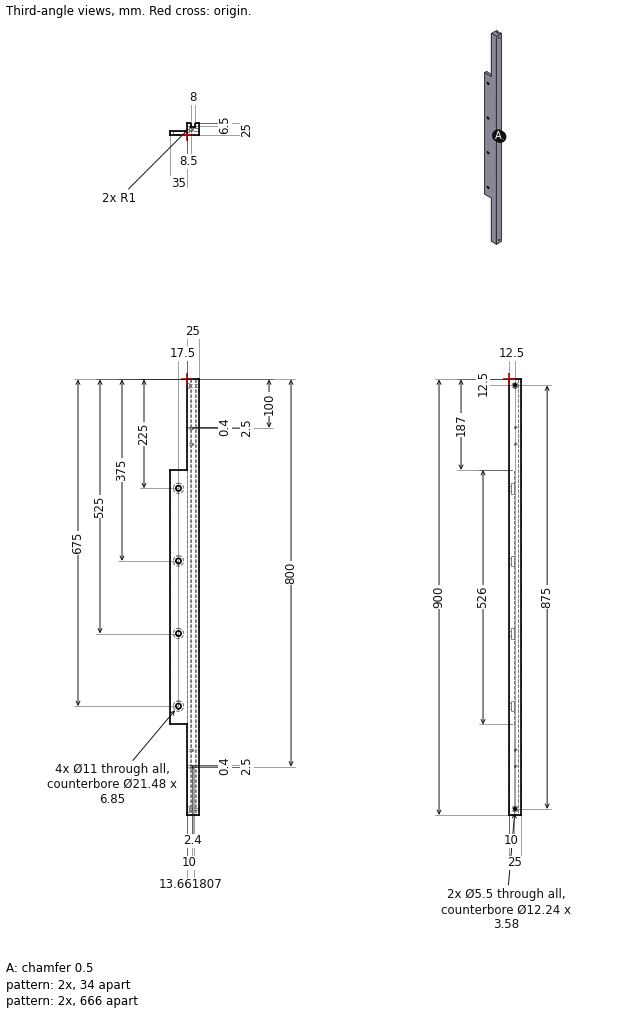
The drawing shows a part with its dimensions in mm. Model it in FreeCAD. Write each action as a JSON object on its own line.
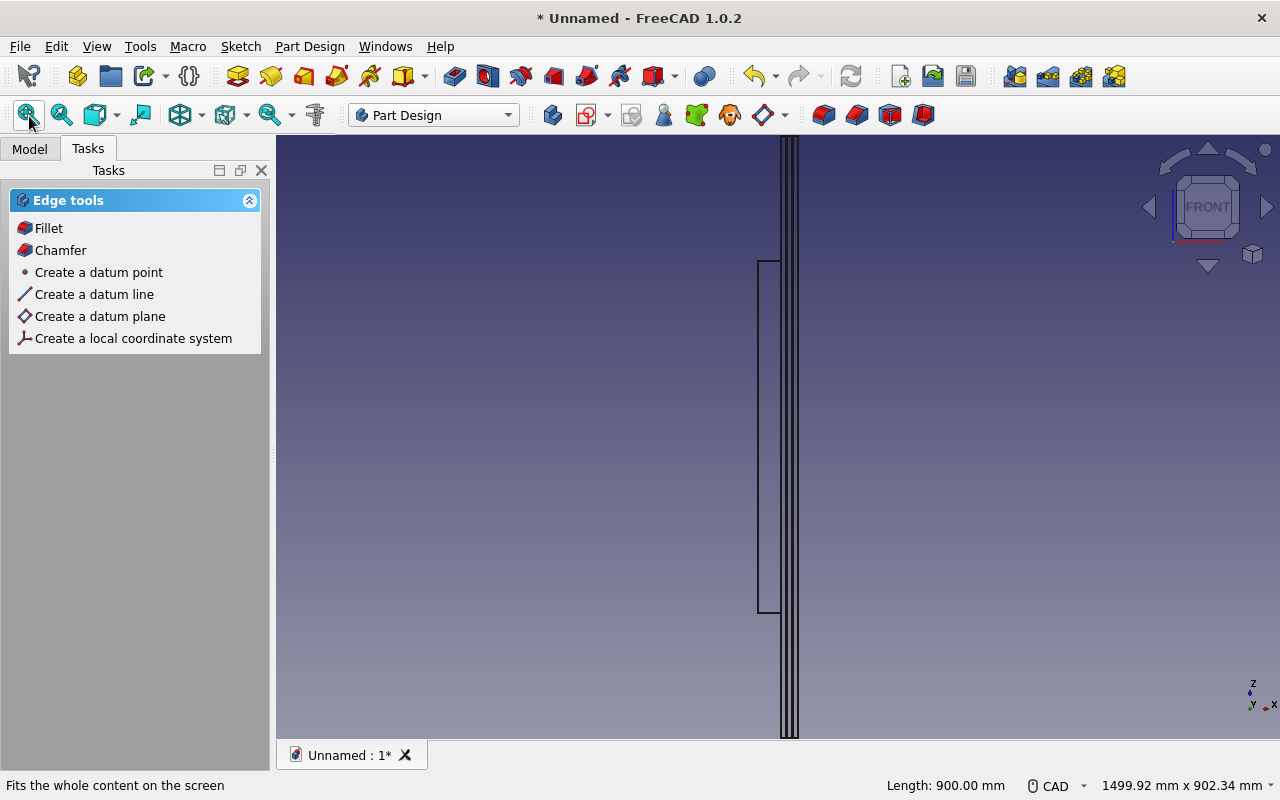
{"action": "key", "text": "3"}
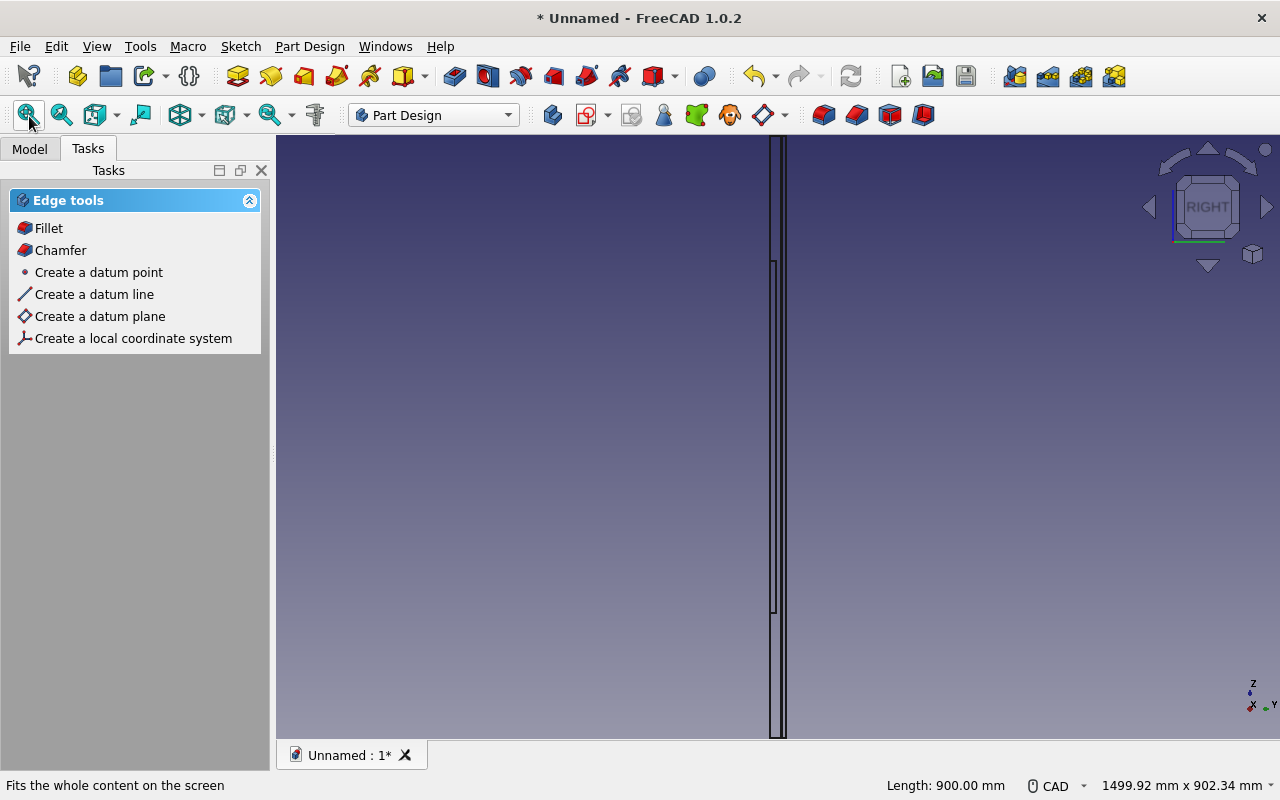
{"action": "scroll", "coordinate": [786, 436], "scroll_direction": "up", "scroll_amount": 6}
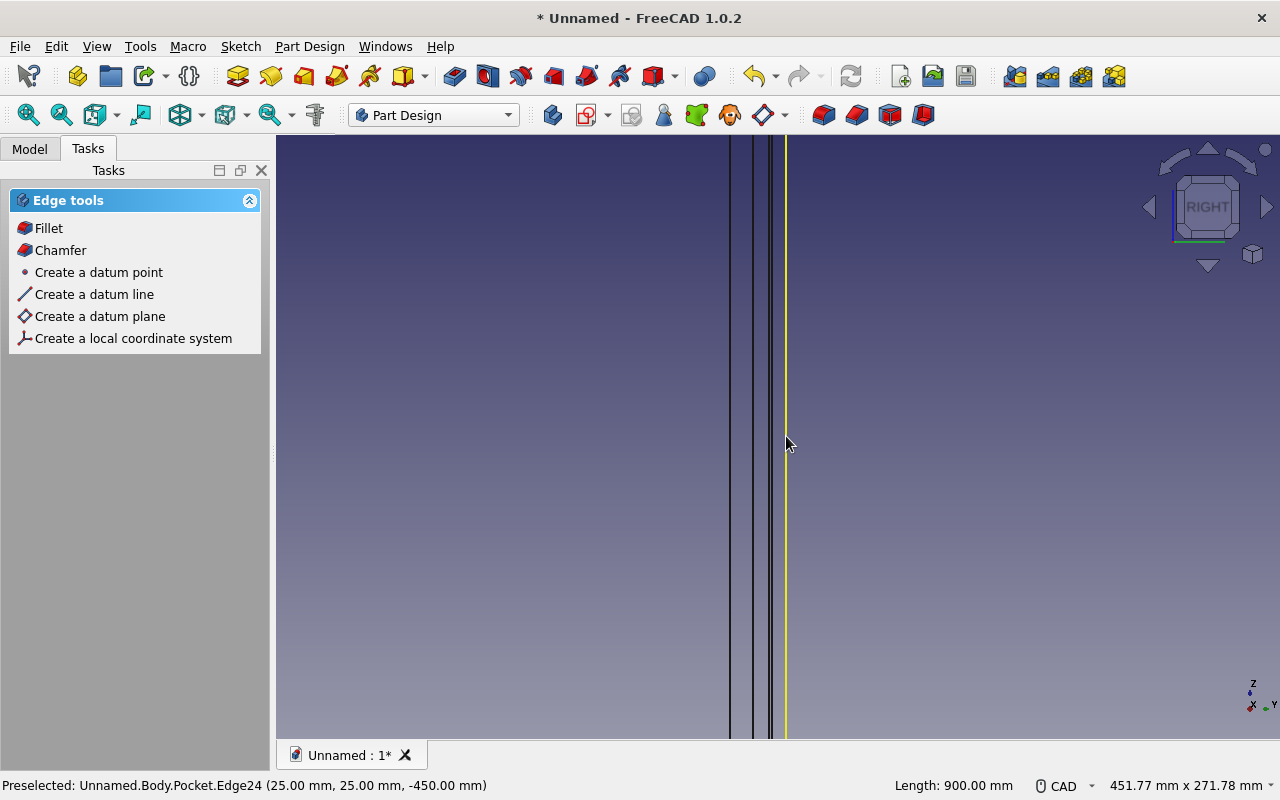
{"action": "left_click", "coordinate": [29, 116]}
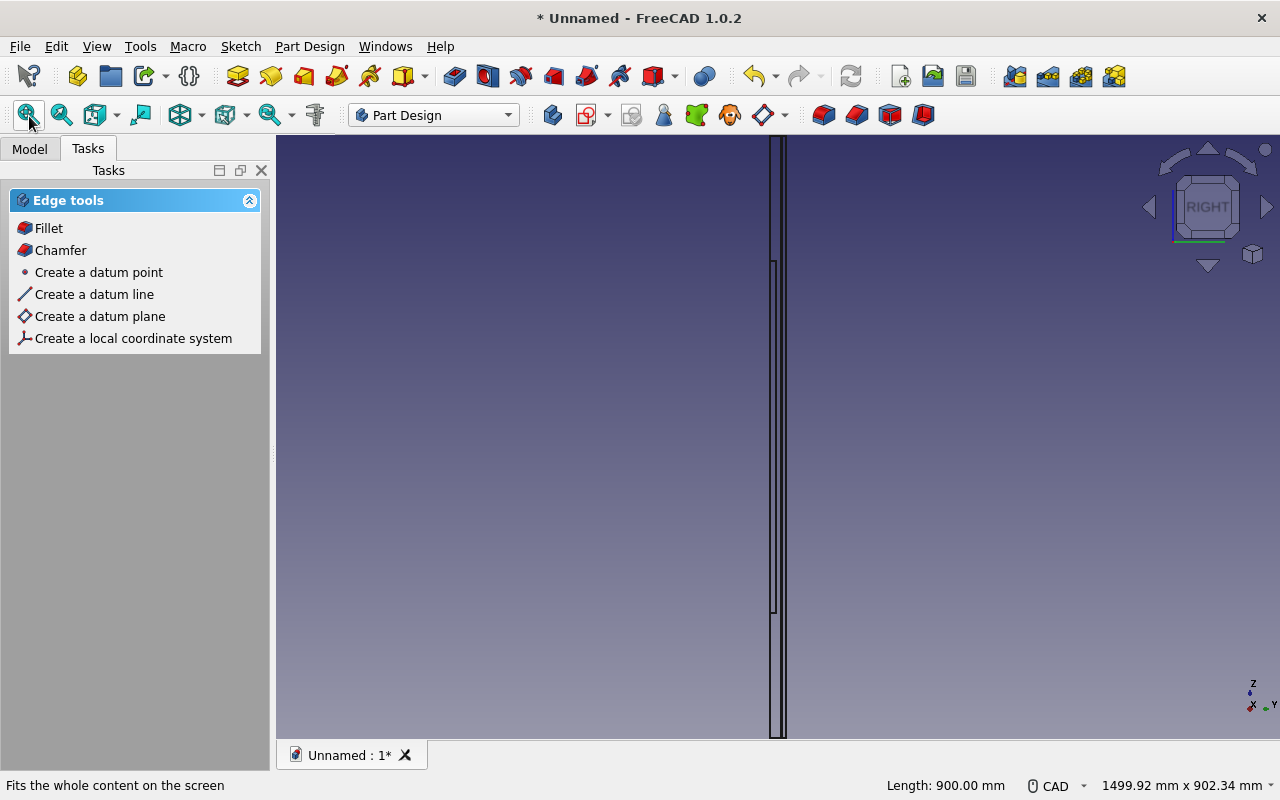
{"action": "key", "text": "5"}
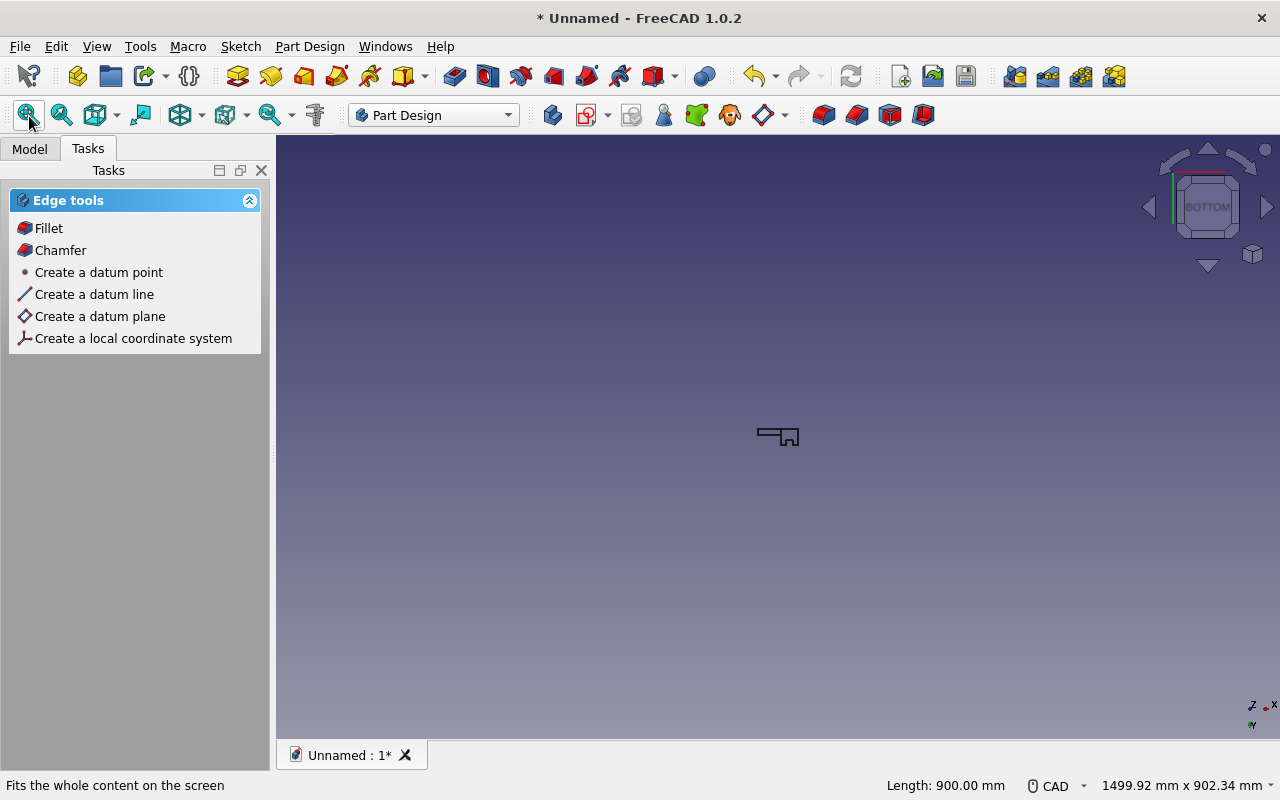
{"action": "left_click", "coordinate": [29, 116]}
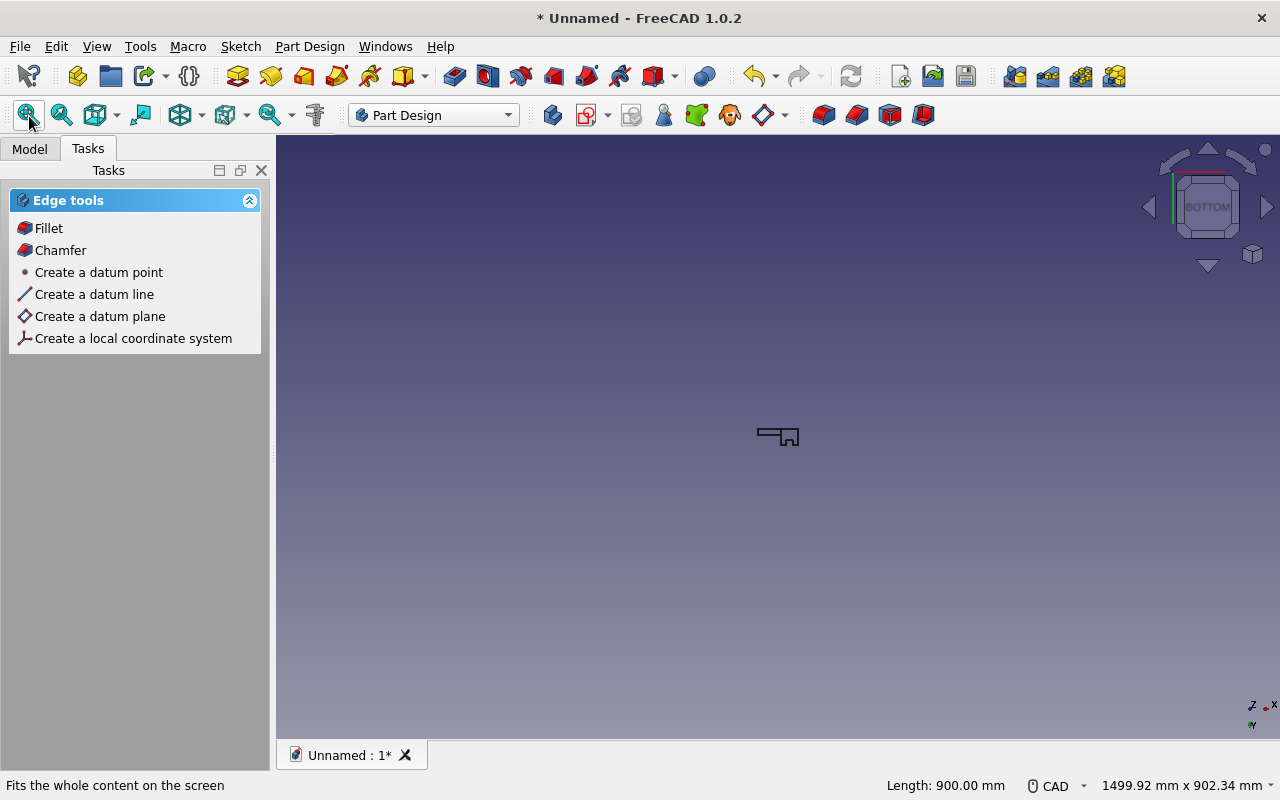
{"action": "scroll", "coordinate": [786, 444], "scroll_direction": "up", "scroll_amount": 6}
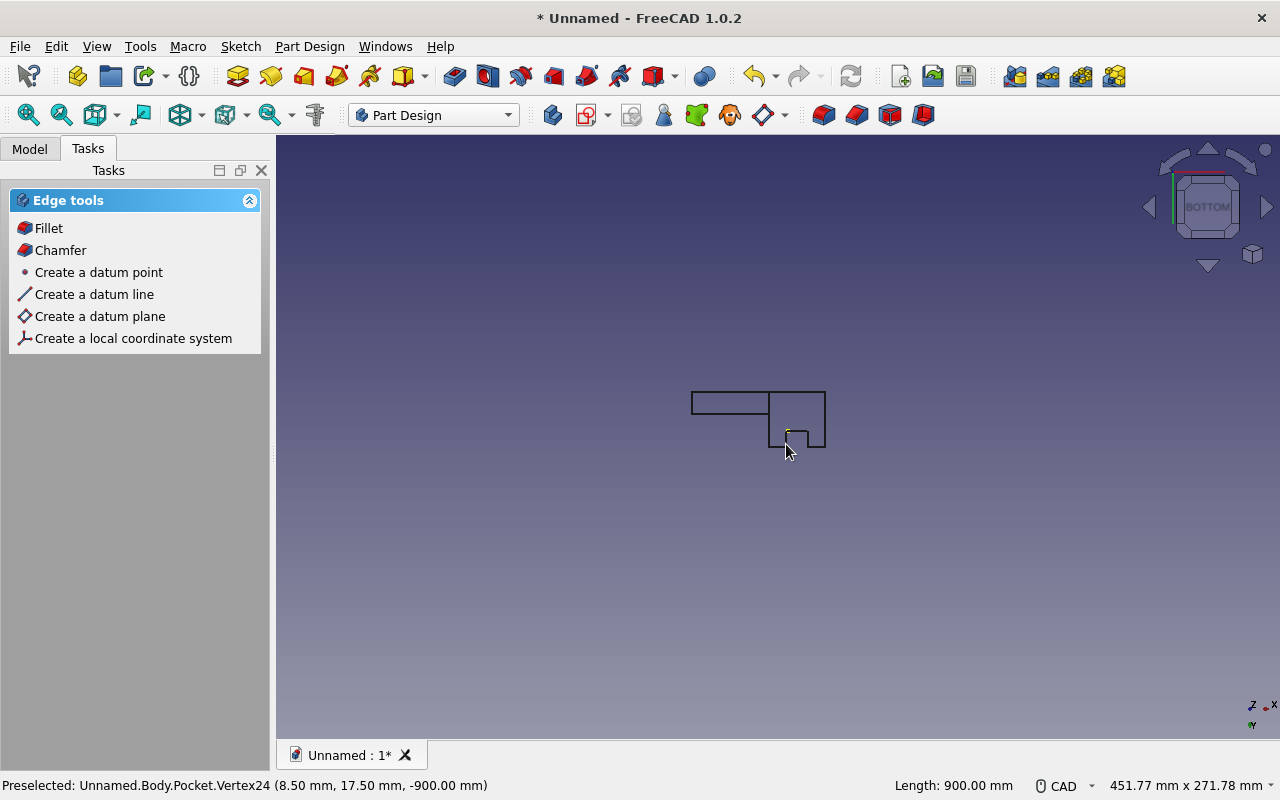
{"action": "left_click", "coordinate": [29, 116]}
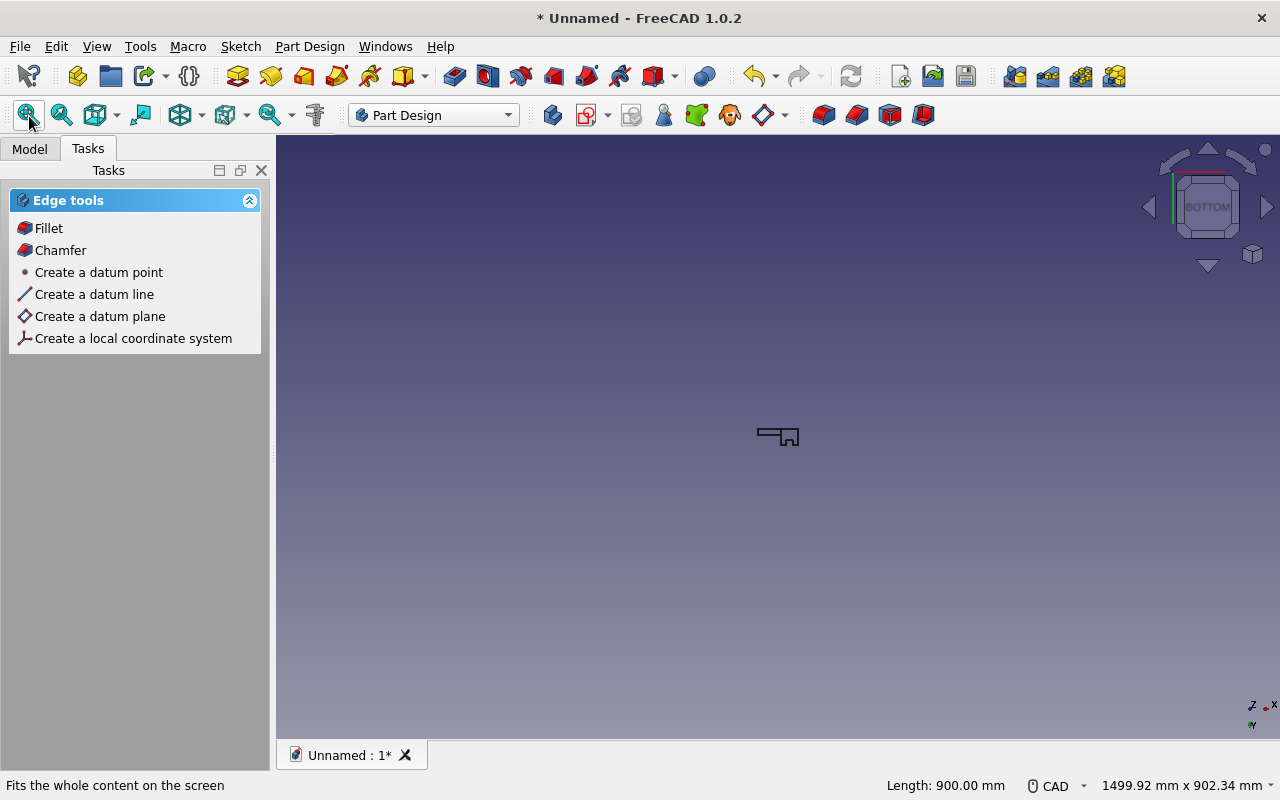
{"action": "key", "text": "4"}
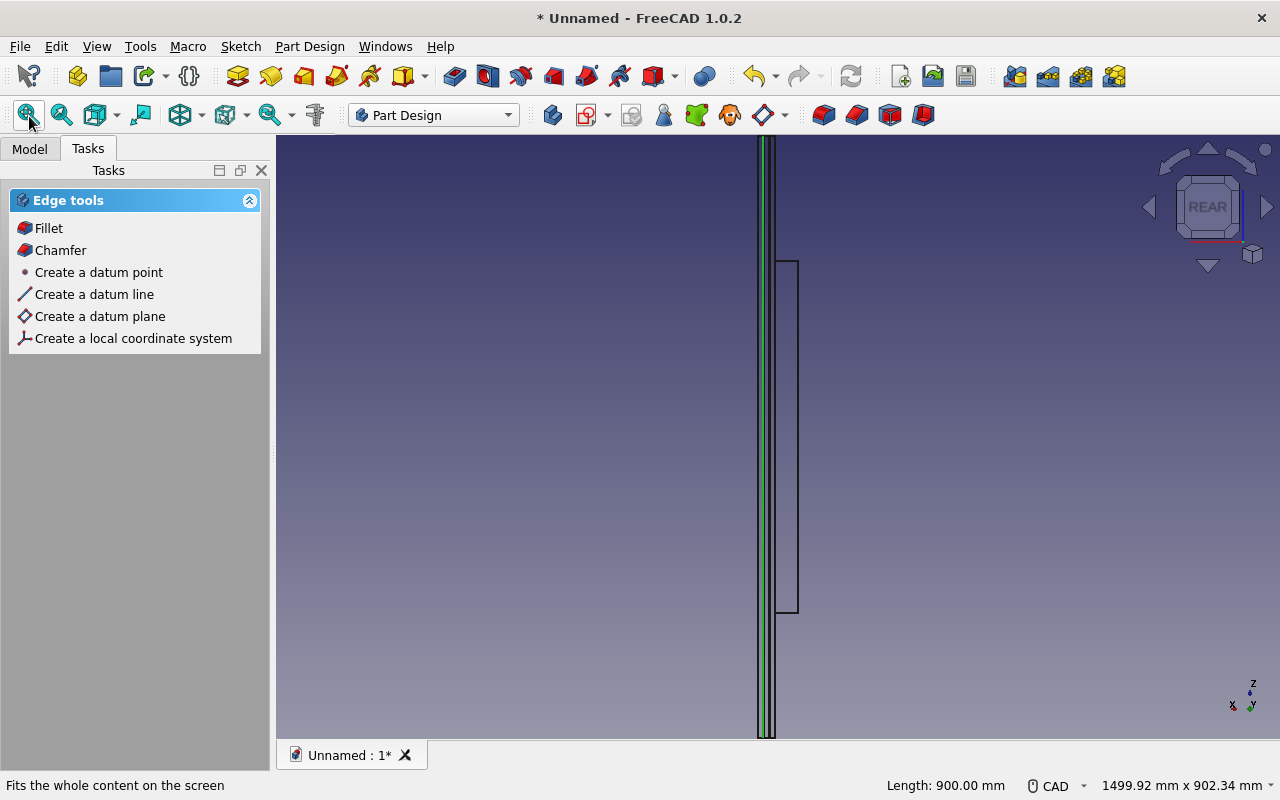
{"action": "scroll", "coordinate": [770, 436], "scroll_direction": "up", "scroll_amount": 6}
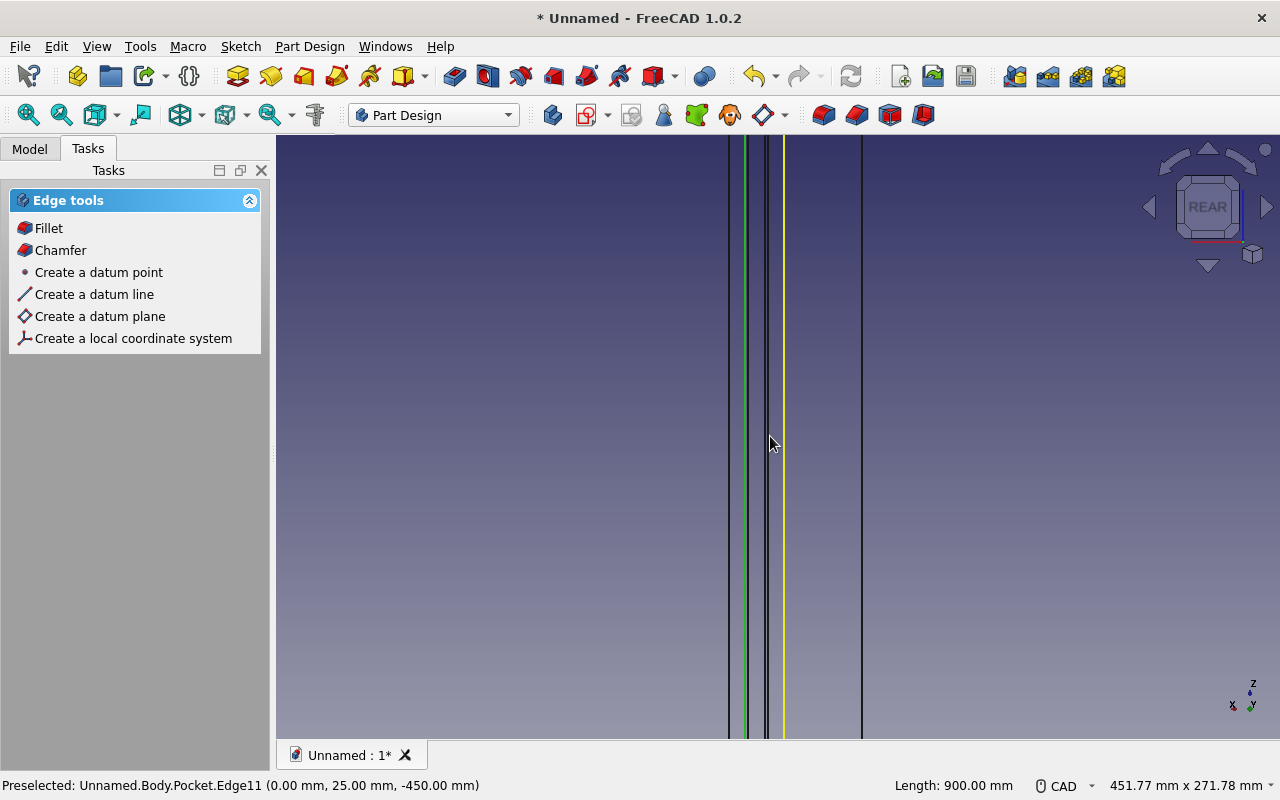
{"action": "left_click", "coordinate": [768, 437], "text": "ctrl"}